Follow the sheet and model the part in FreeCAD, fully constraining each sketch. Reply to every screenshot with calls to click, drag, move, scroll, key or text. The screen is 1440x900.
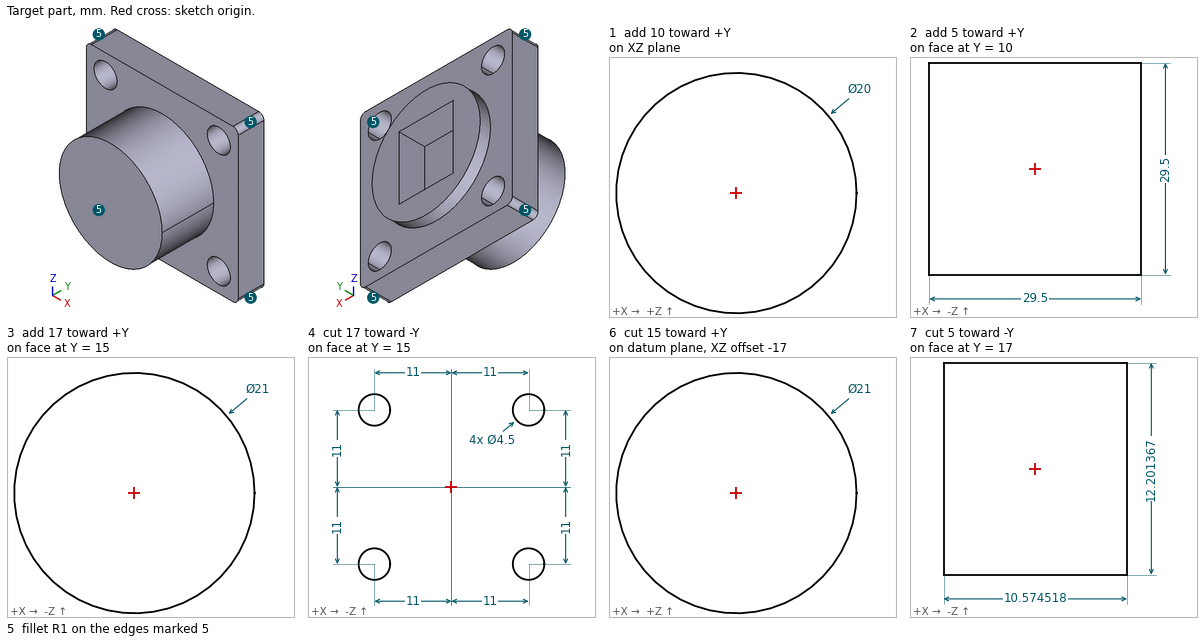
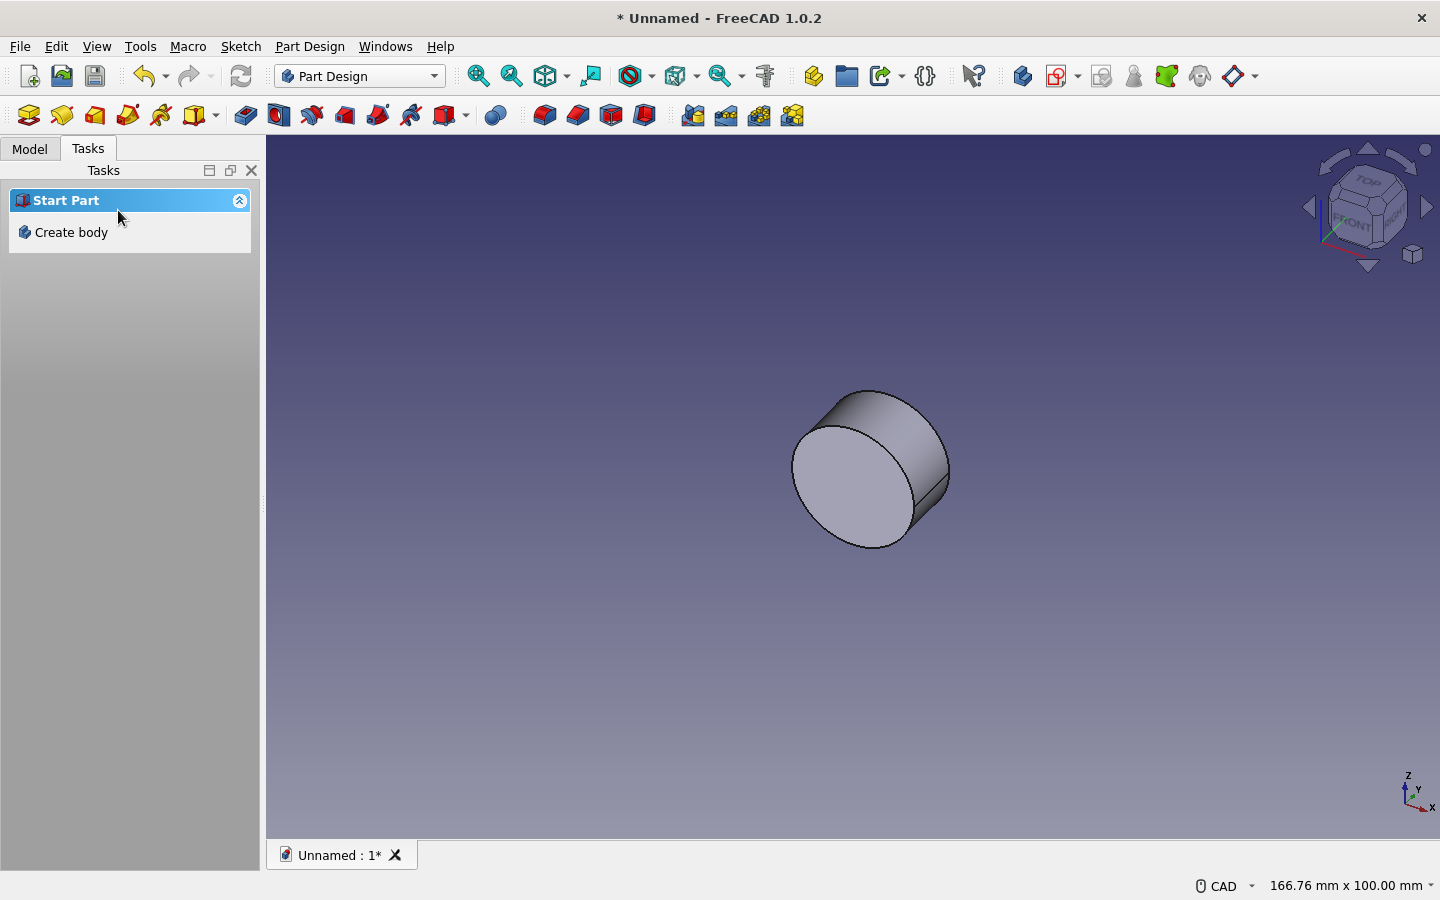
click(479, 76)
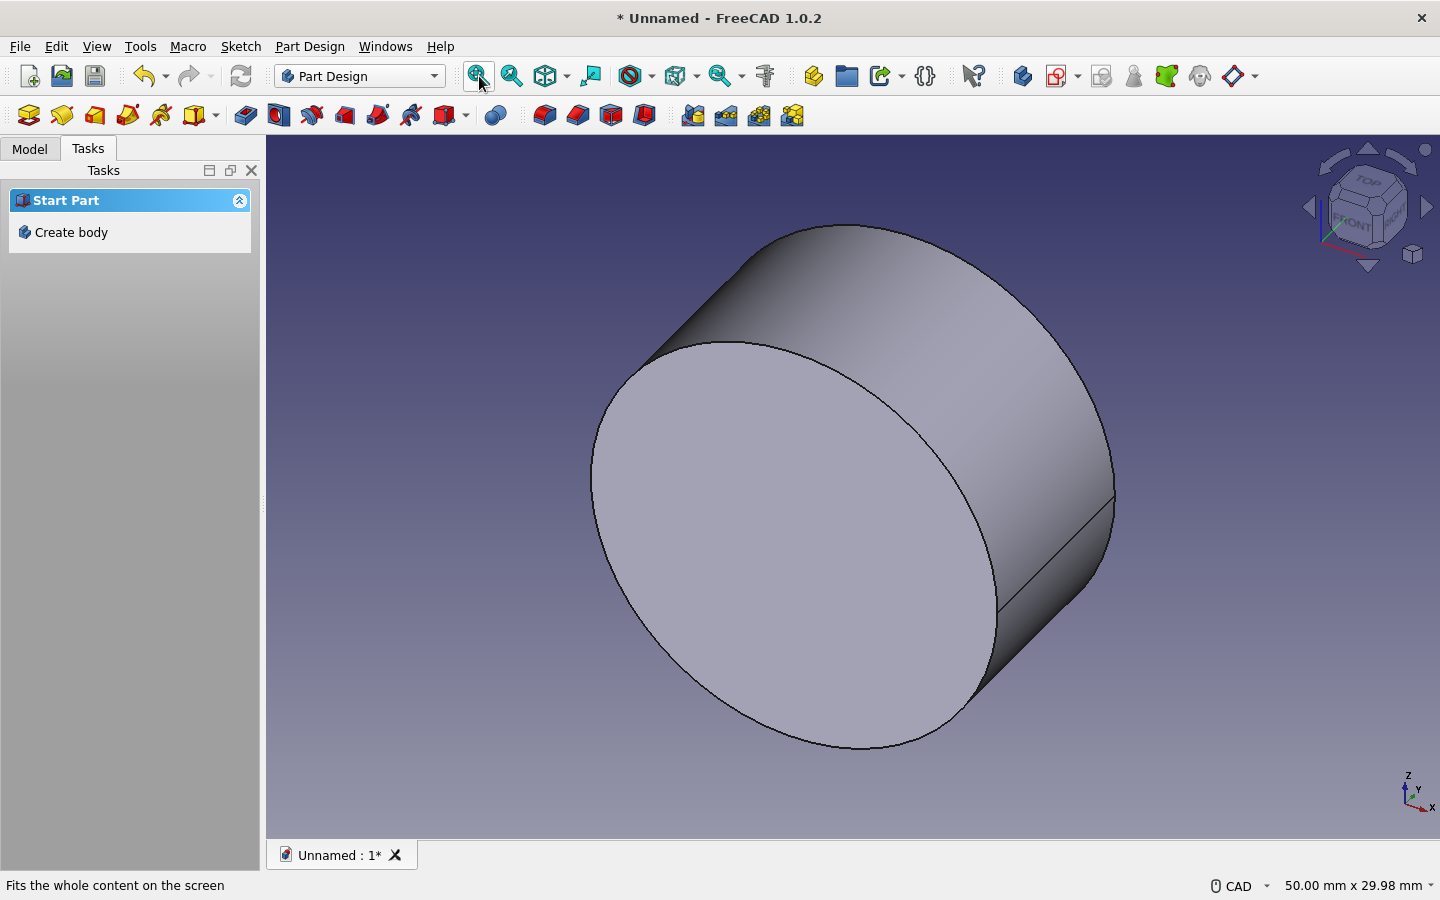
key(4)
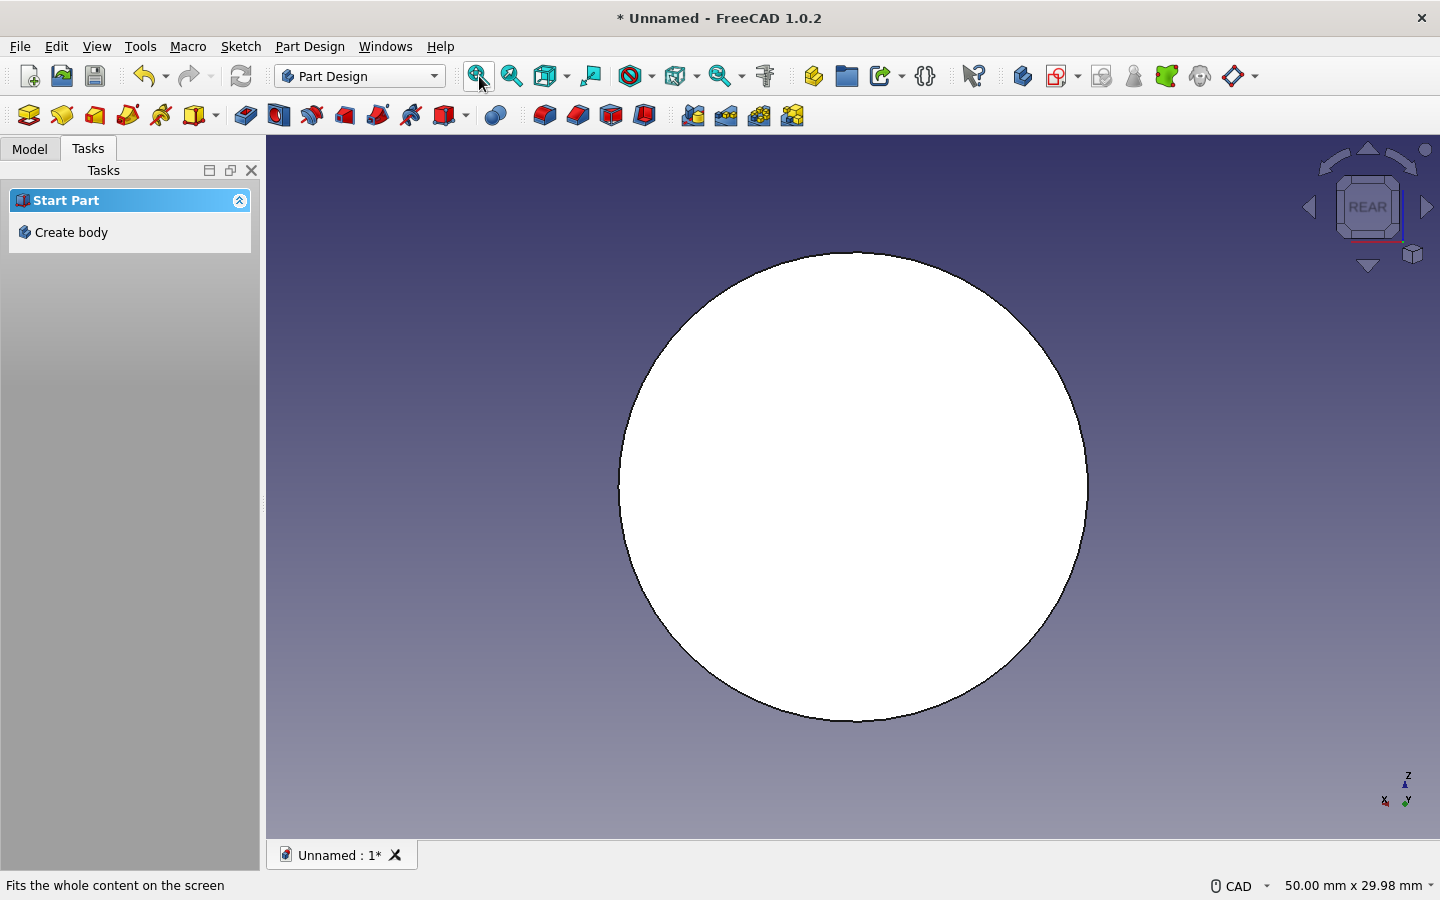
click(853, 486)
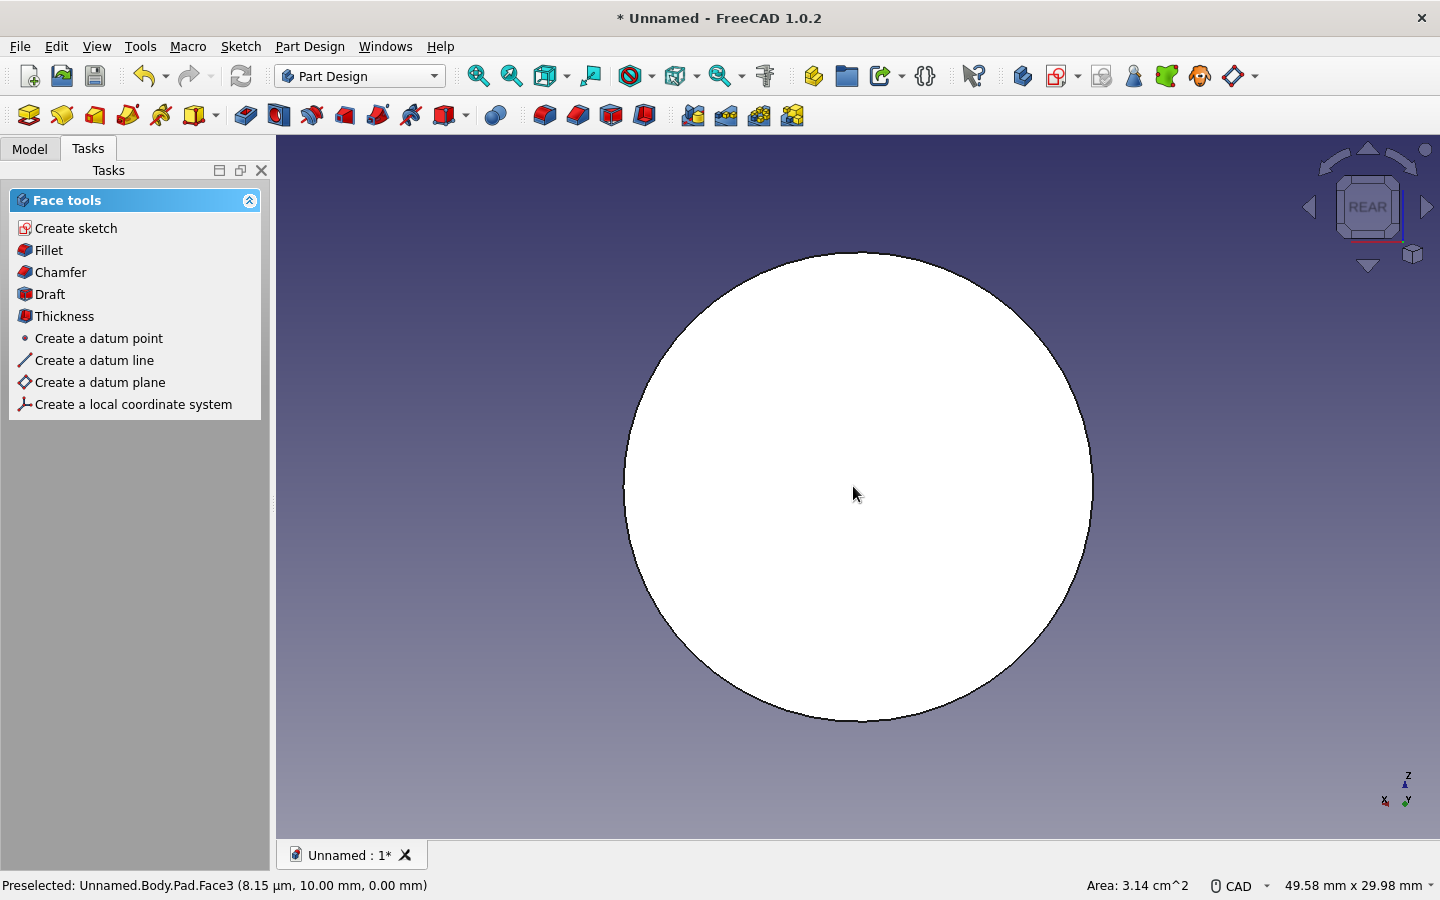
click(1056, 76)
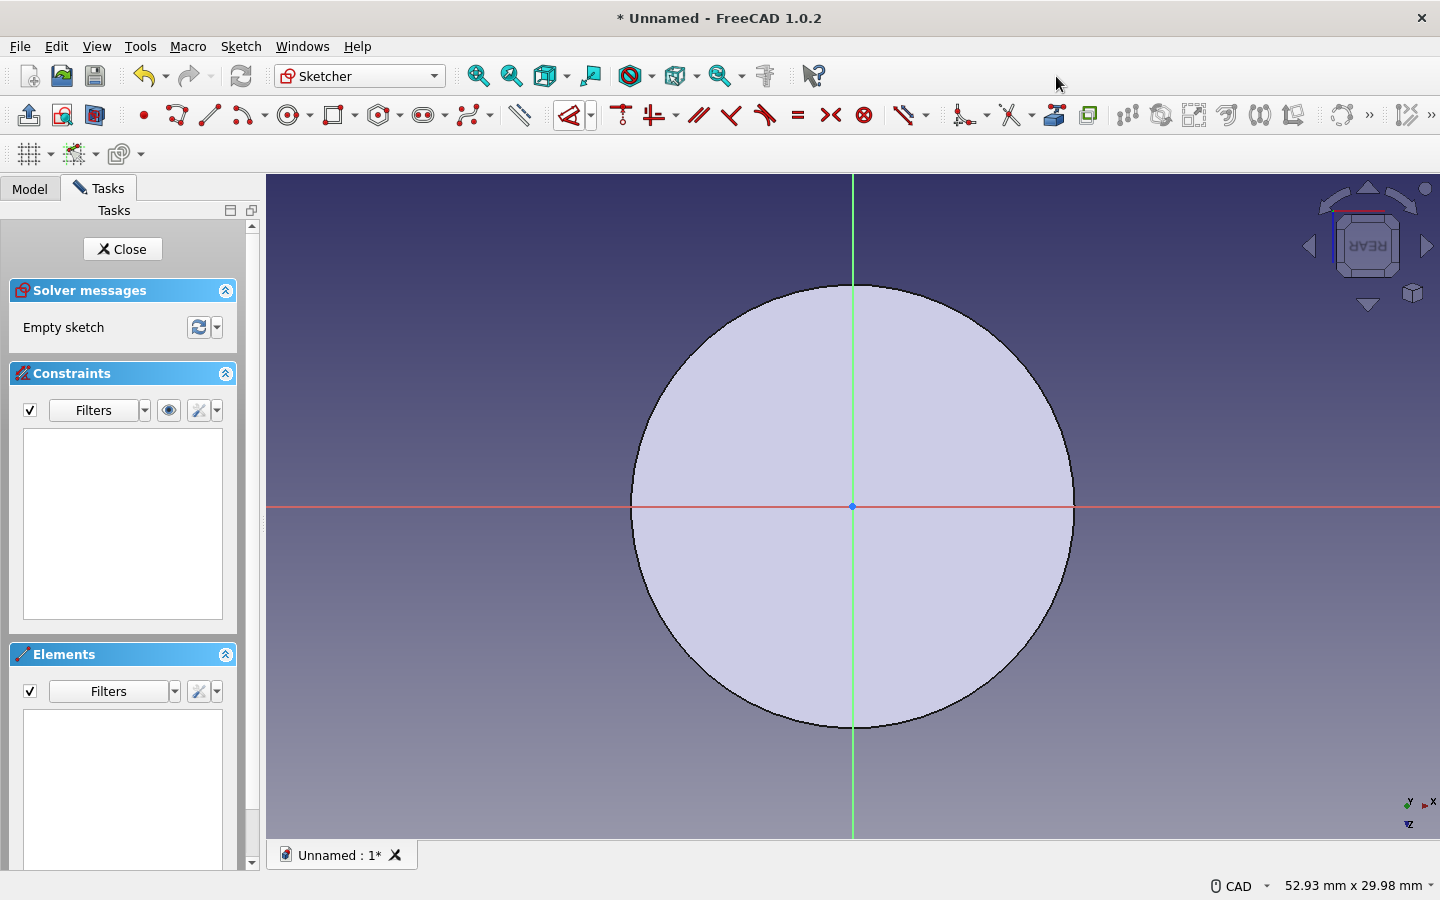
scroll(646, 507, down, 2)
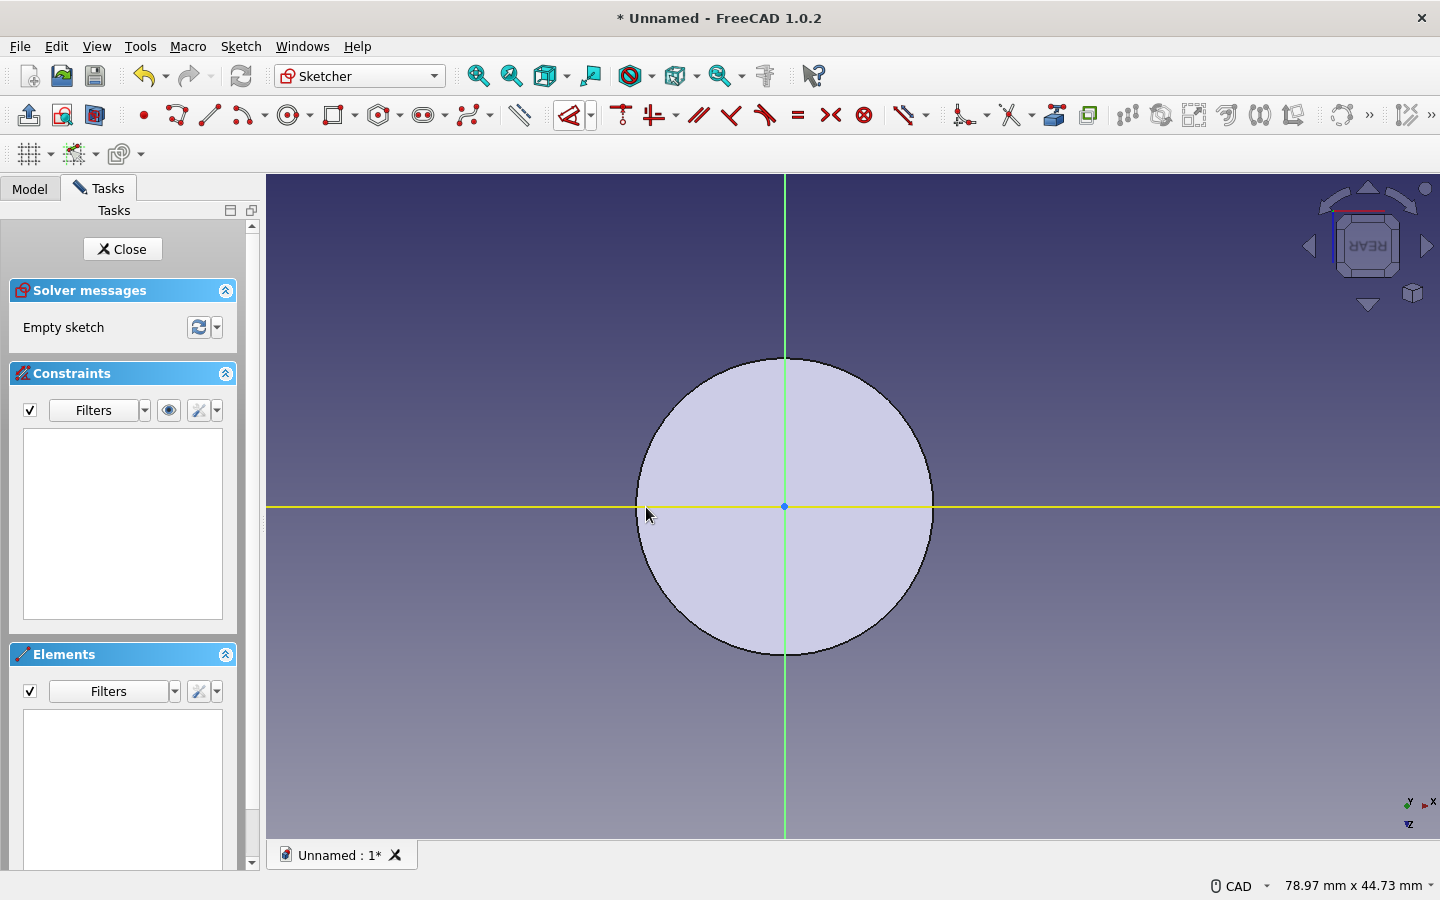
click(354, 116)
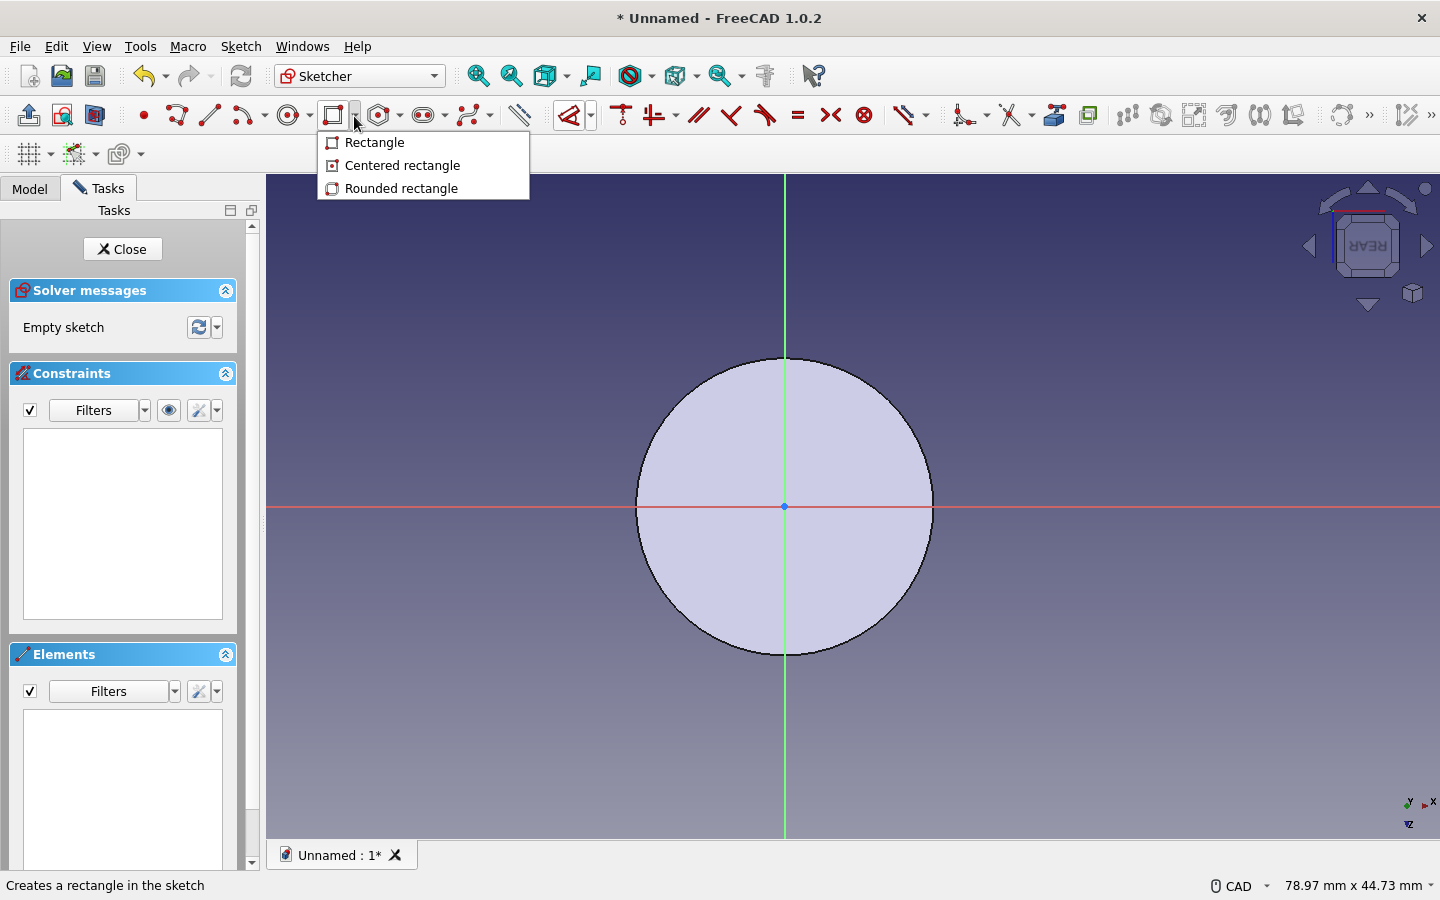
click(424, 166)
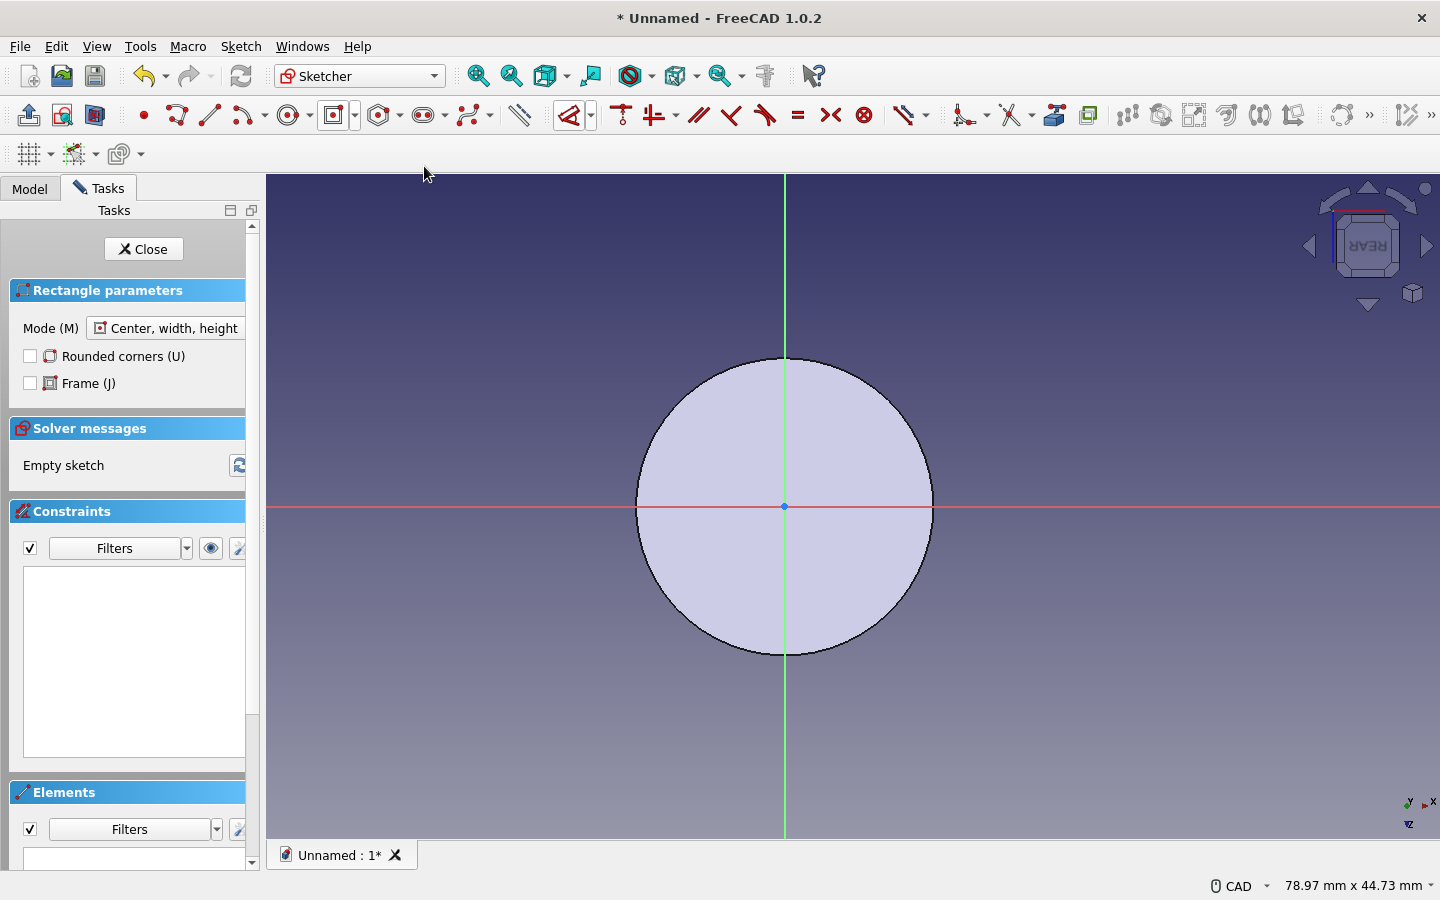
click(785, 507)
click(1004, 288)
key(Escape)